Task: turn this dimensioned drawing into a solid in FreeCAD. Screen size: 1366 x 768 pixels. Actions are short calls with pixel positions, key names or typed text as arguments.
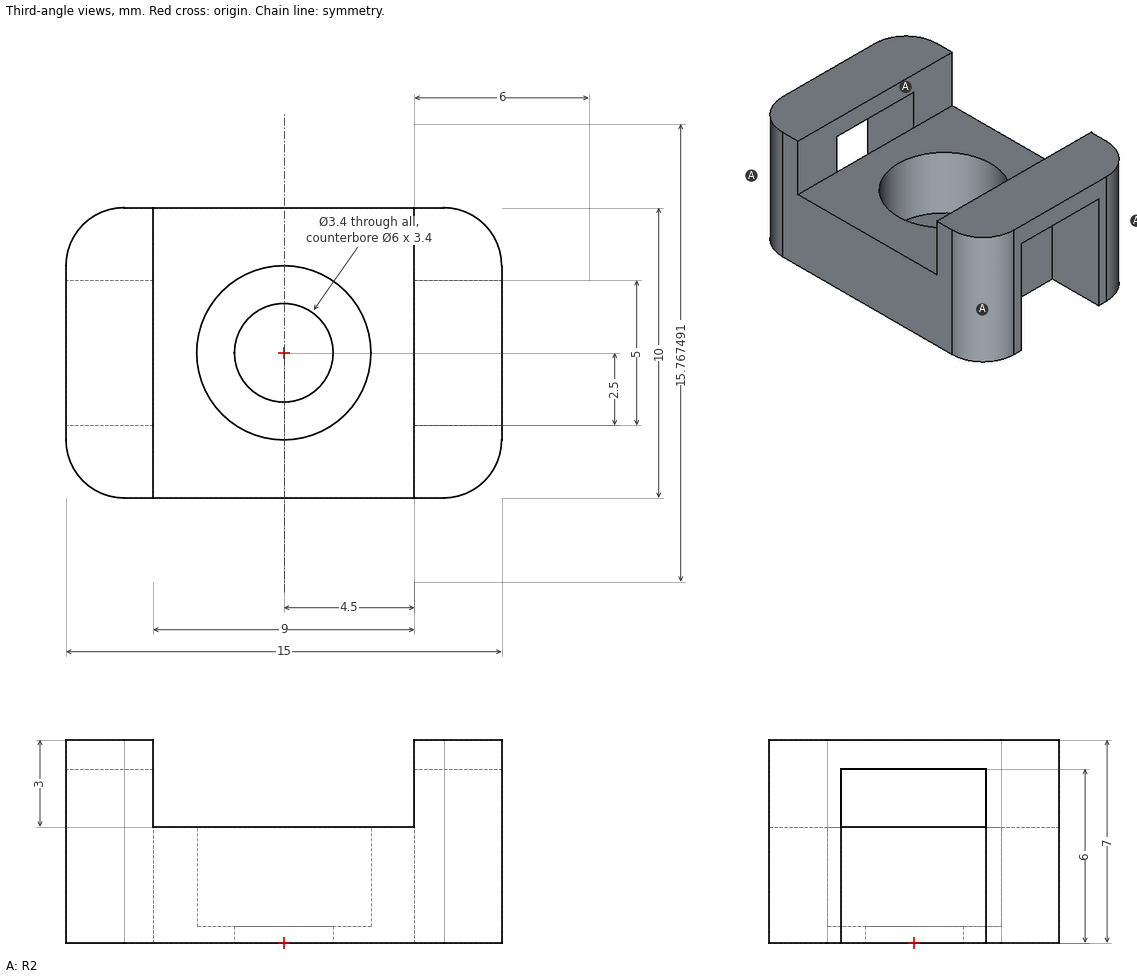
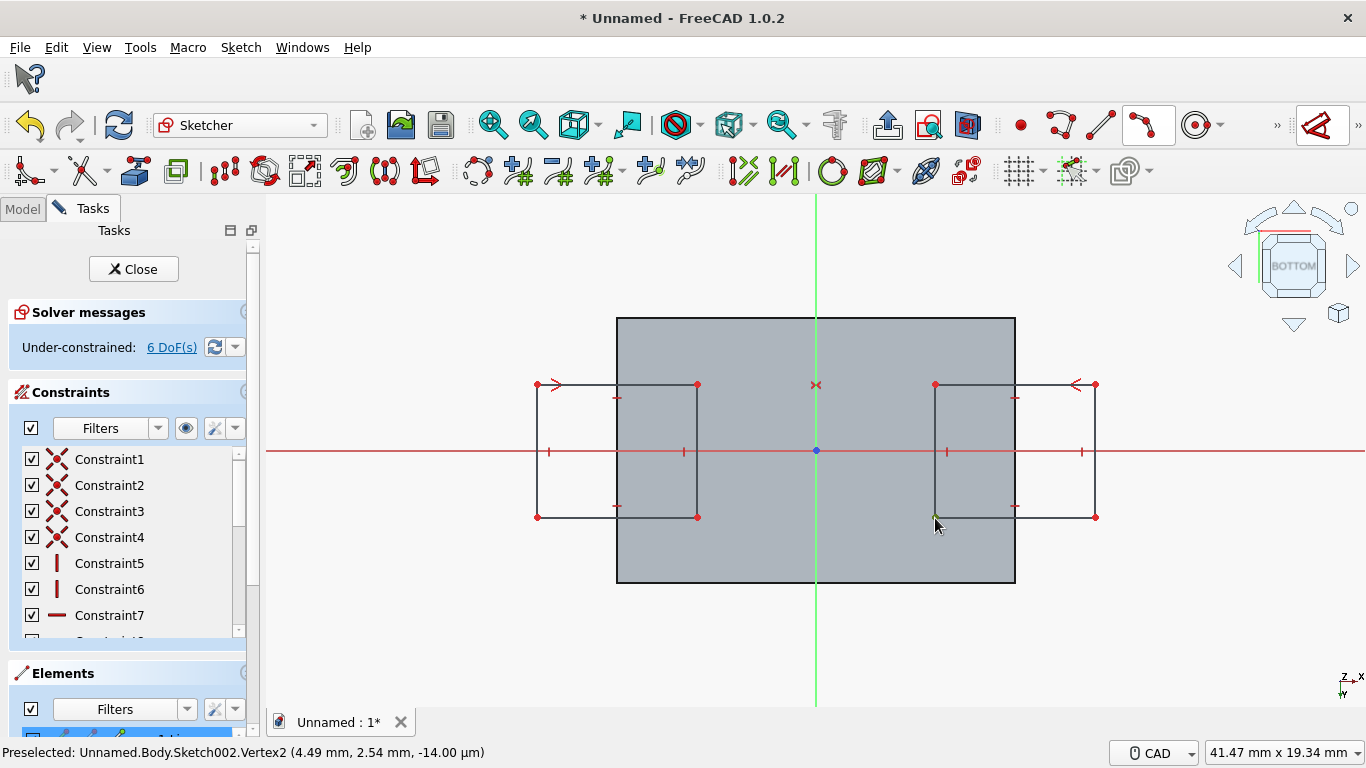
click(697, 518)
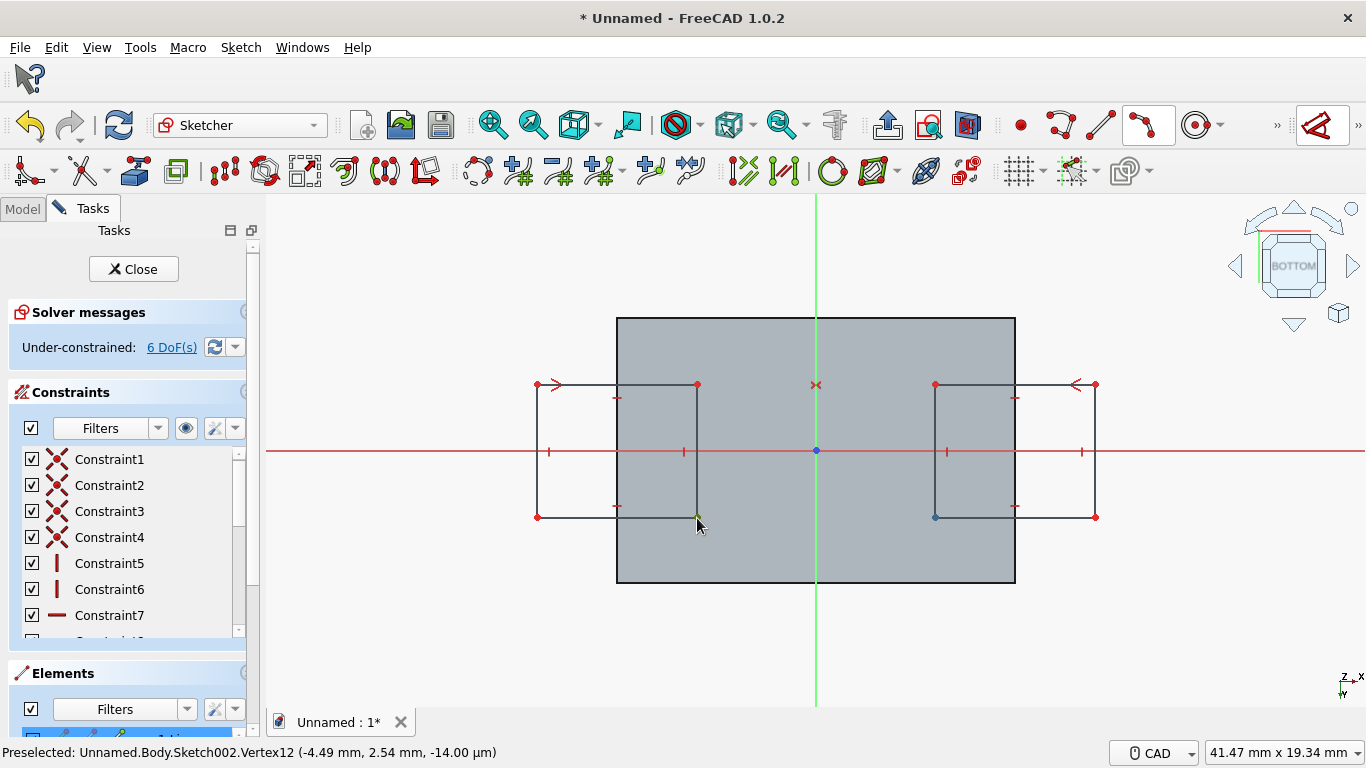
click(816, 646)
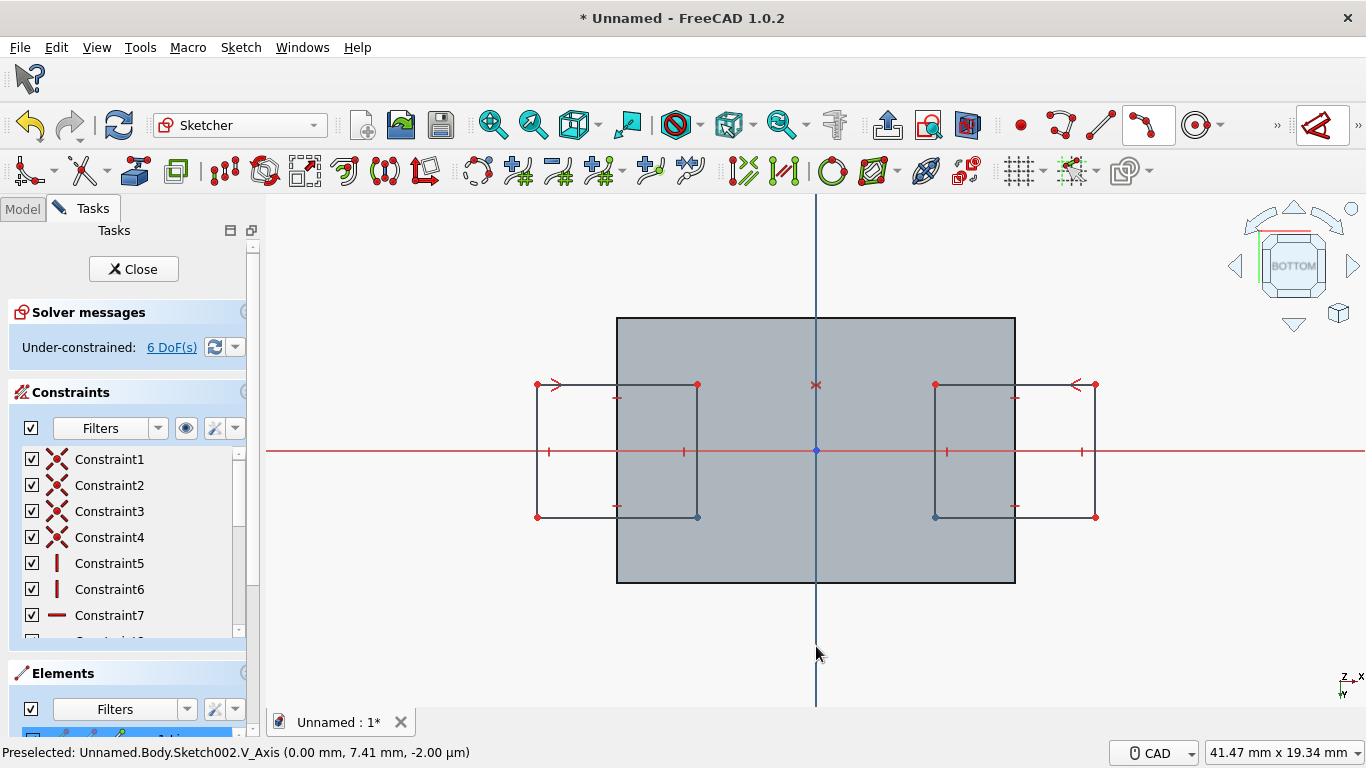
key(s)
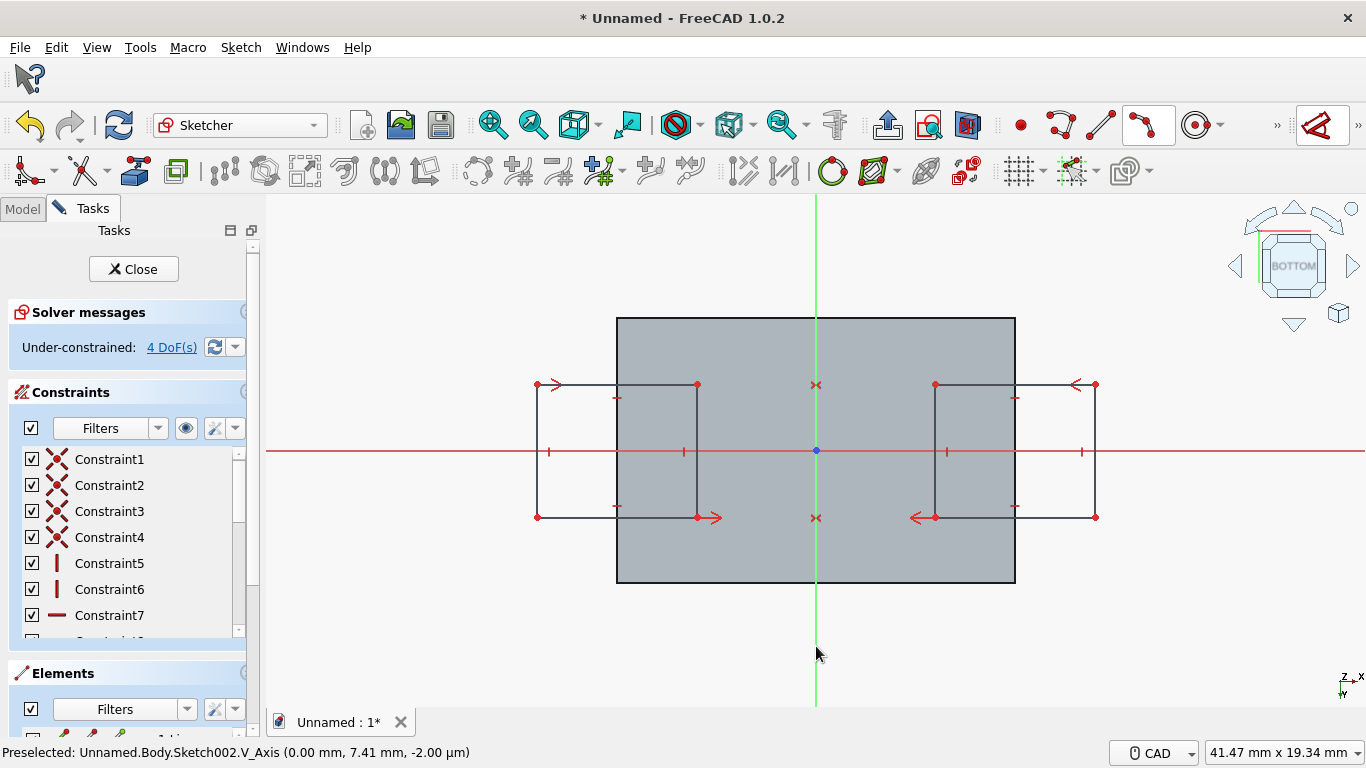
click(935, 425)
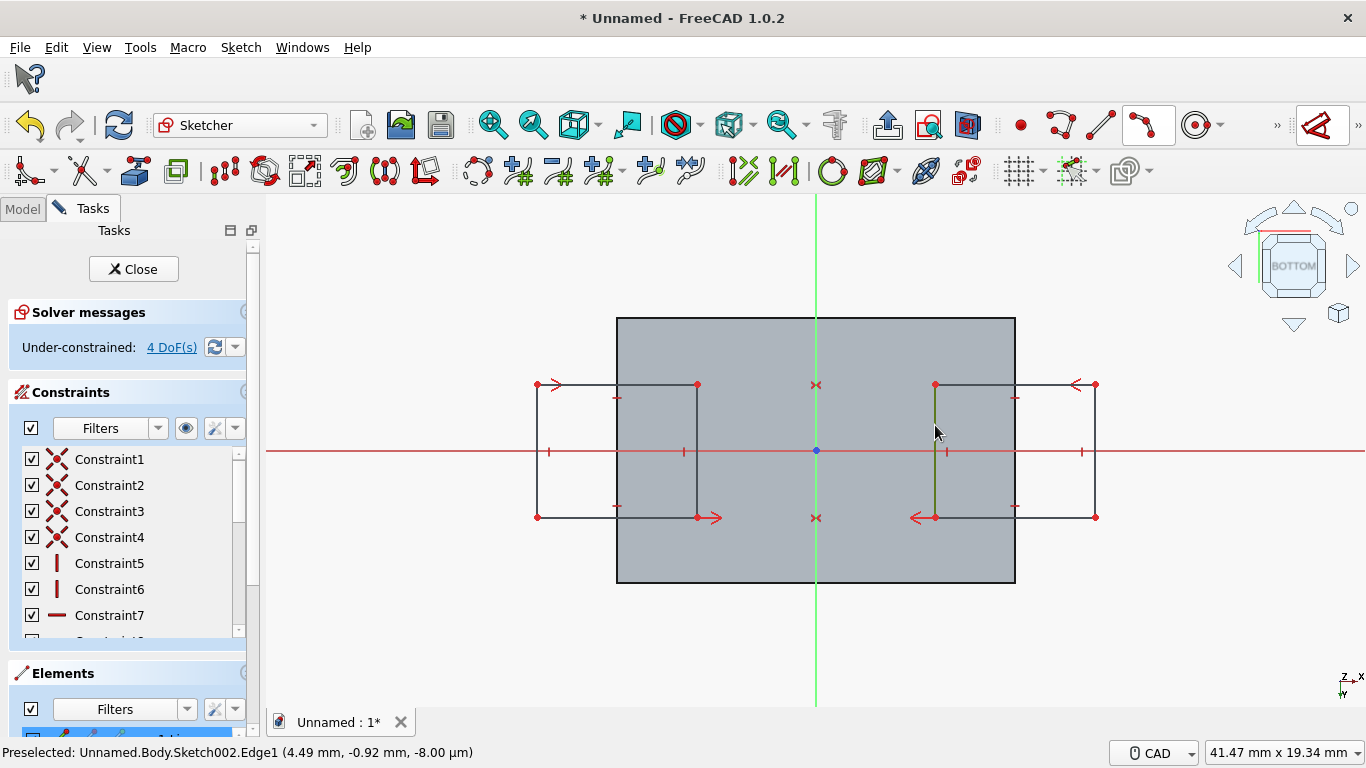
key(i)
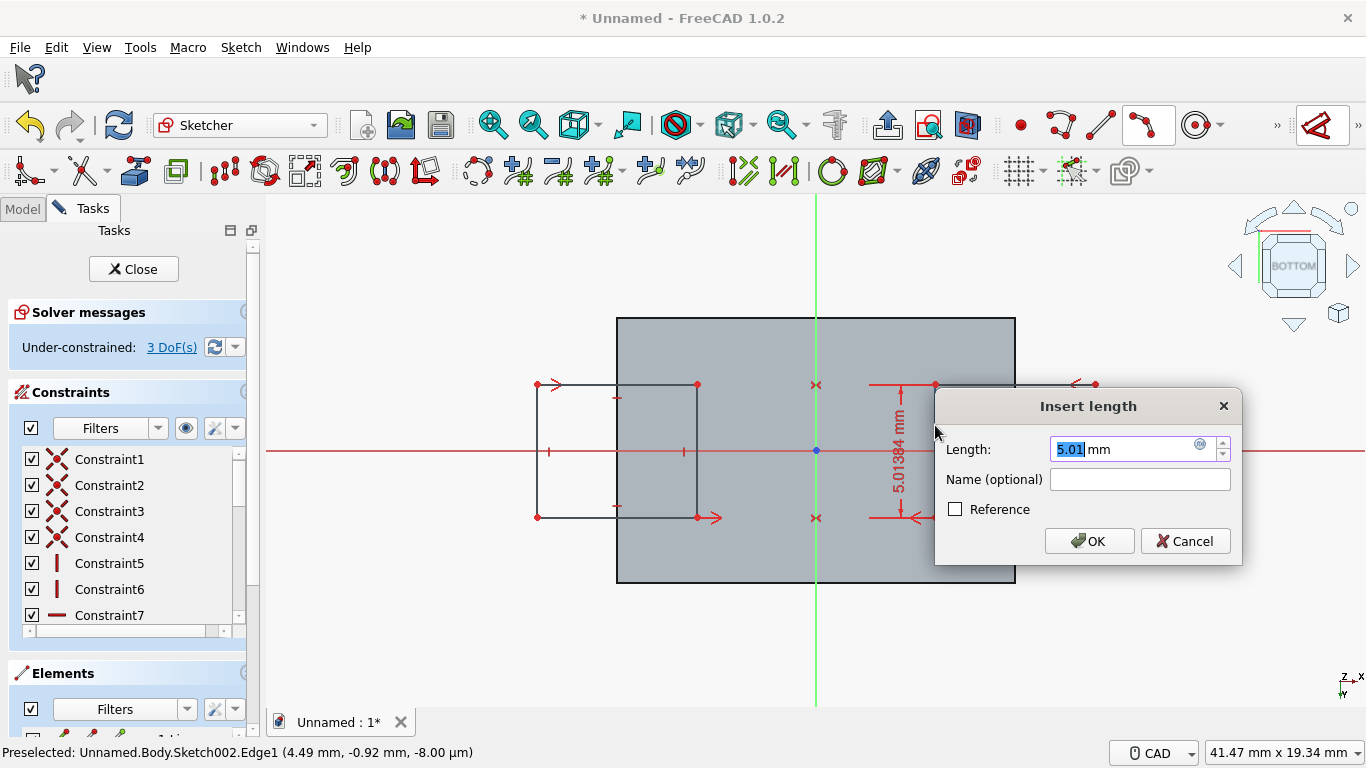
text(5)
key(Return)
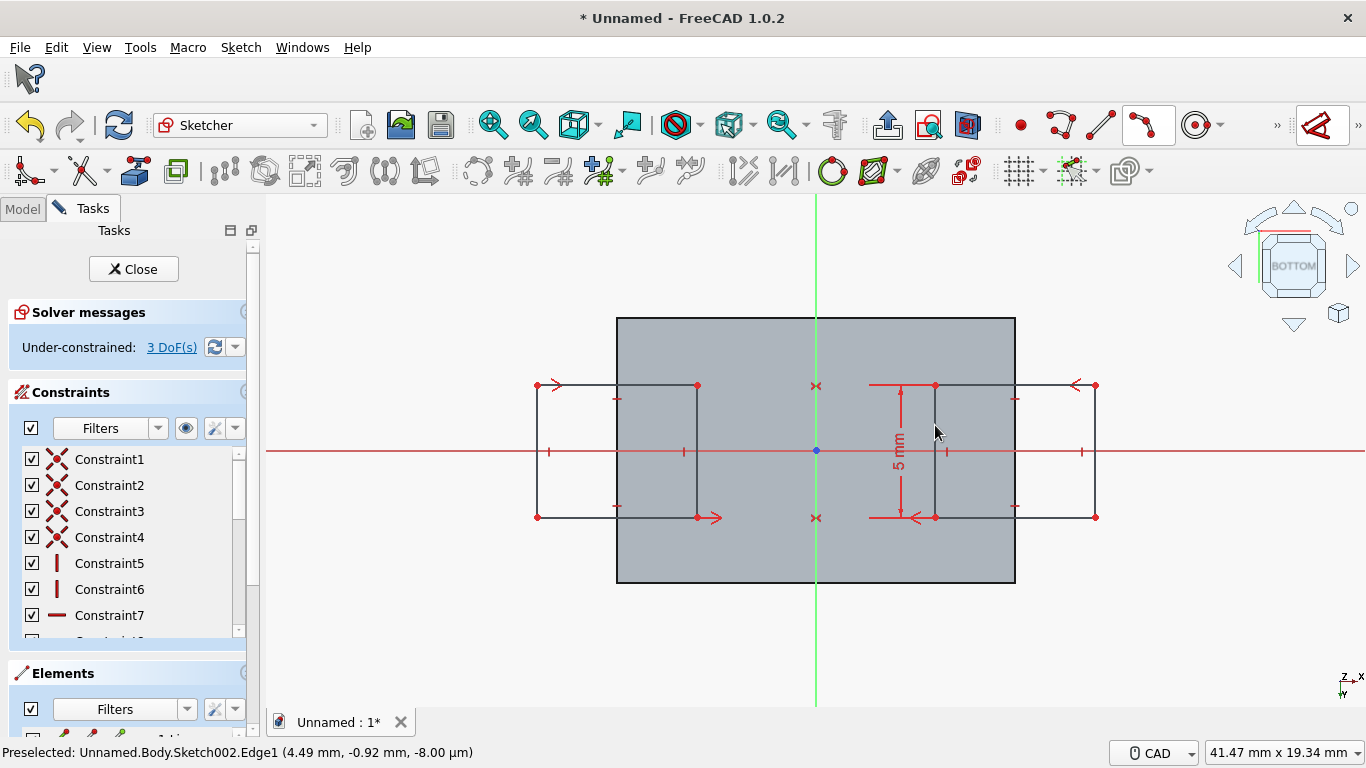
click(983, 518)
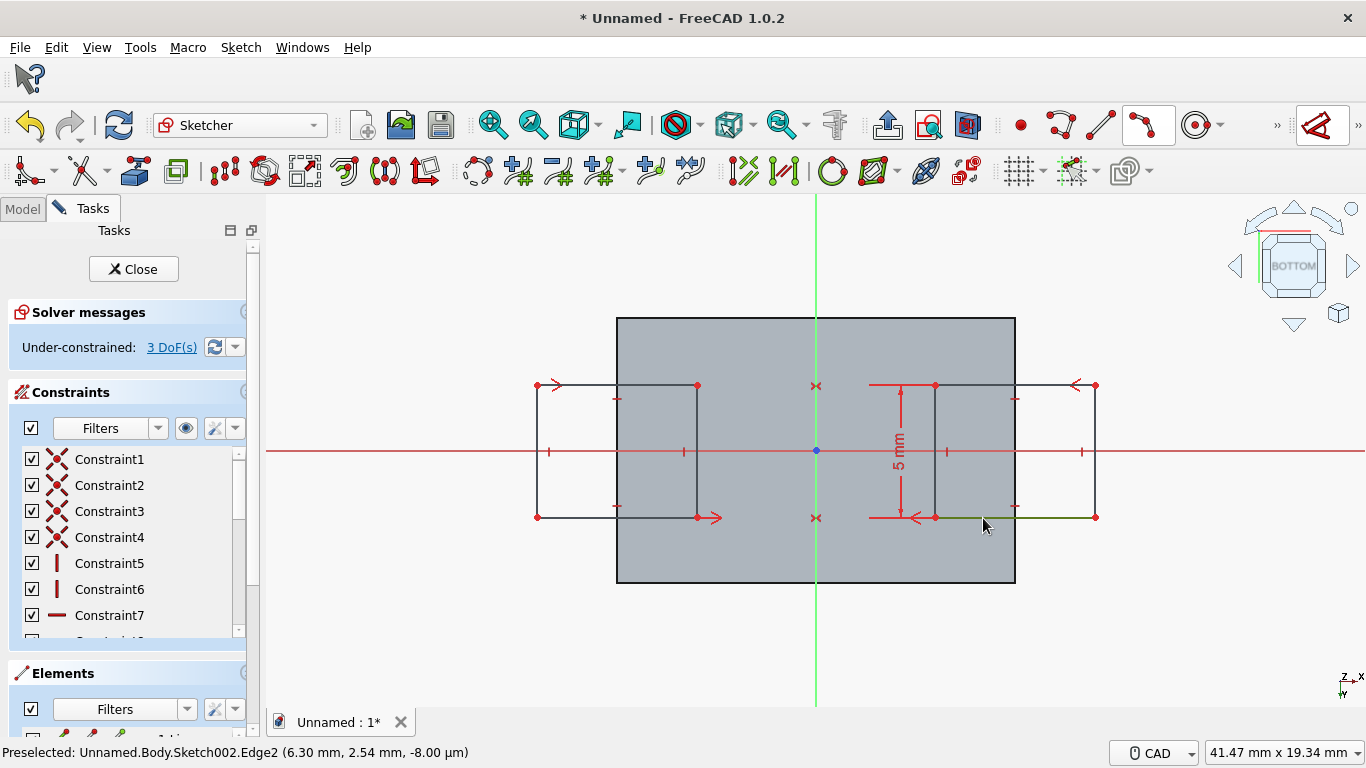
click(1344, 126)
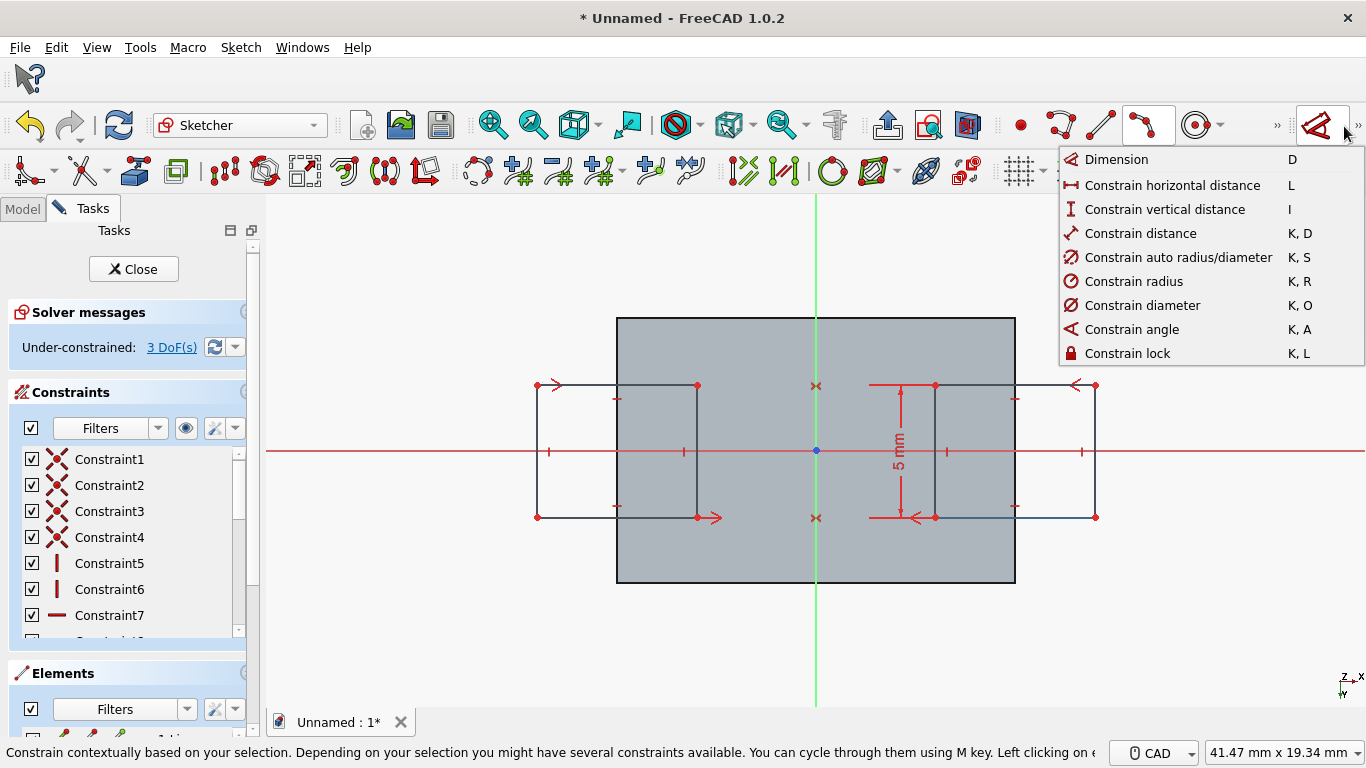
click(1212, 185)